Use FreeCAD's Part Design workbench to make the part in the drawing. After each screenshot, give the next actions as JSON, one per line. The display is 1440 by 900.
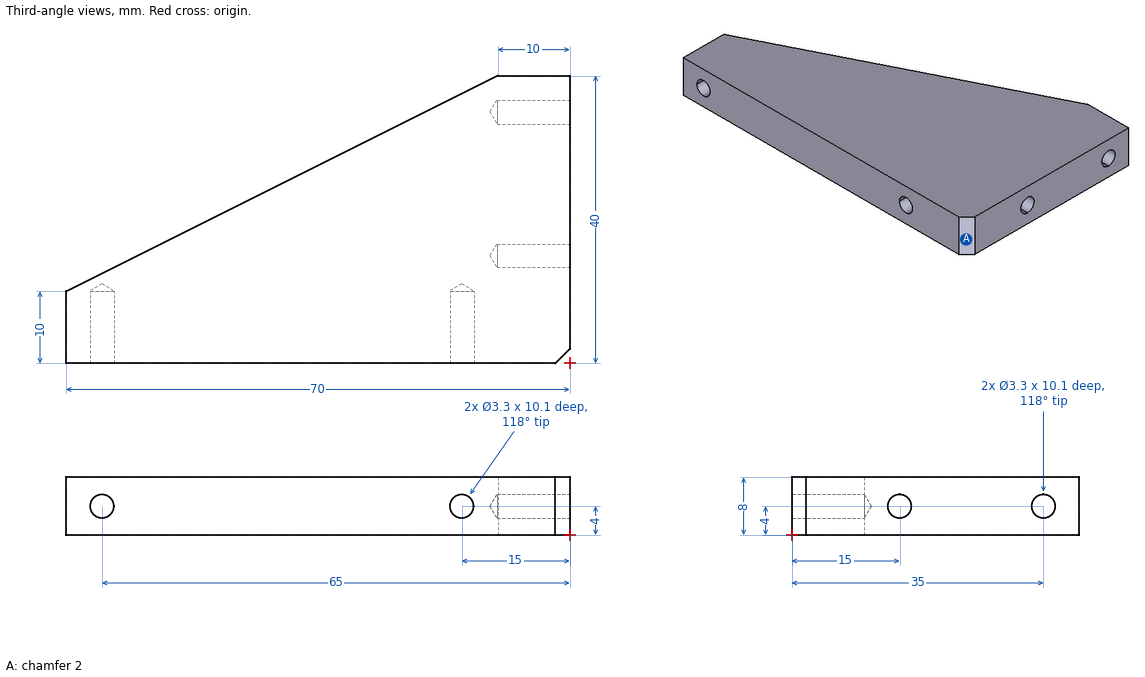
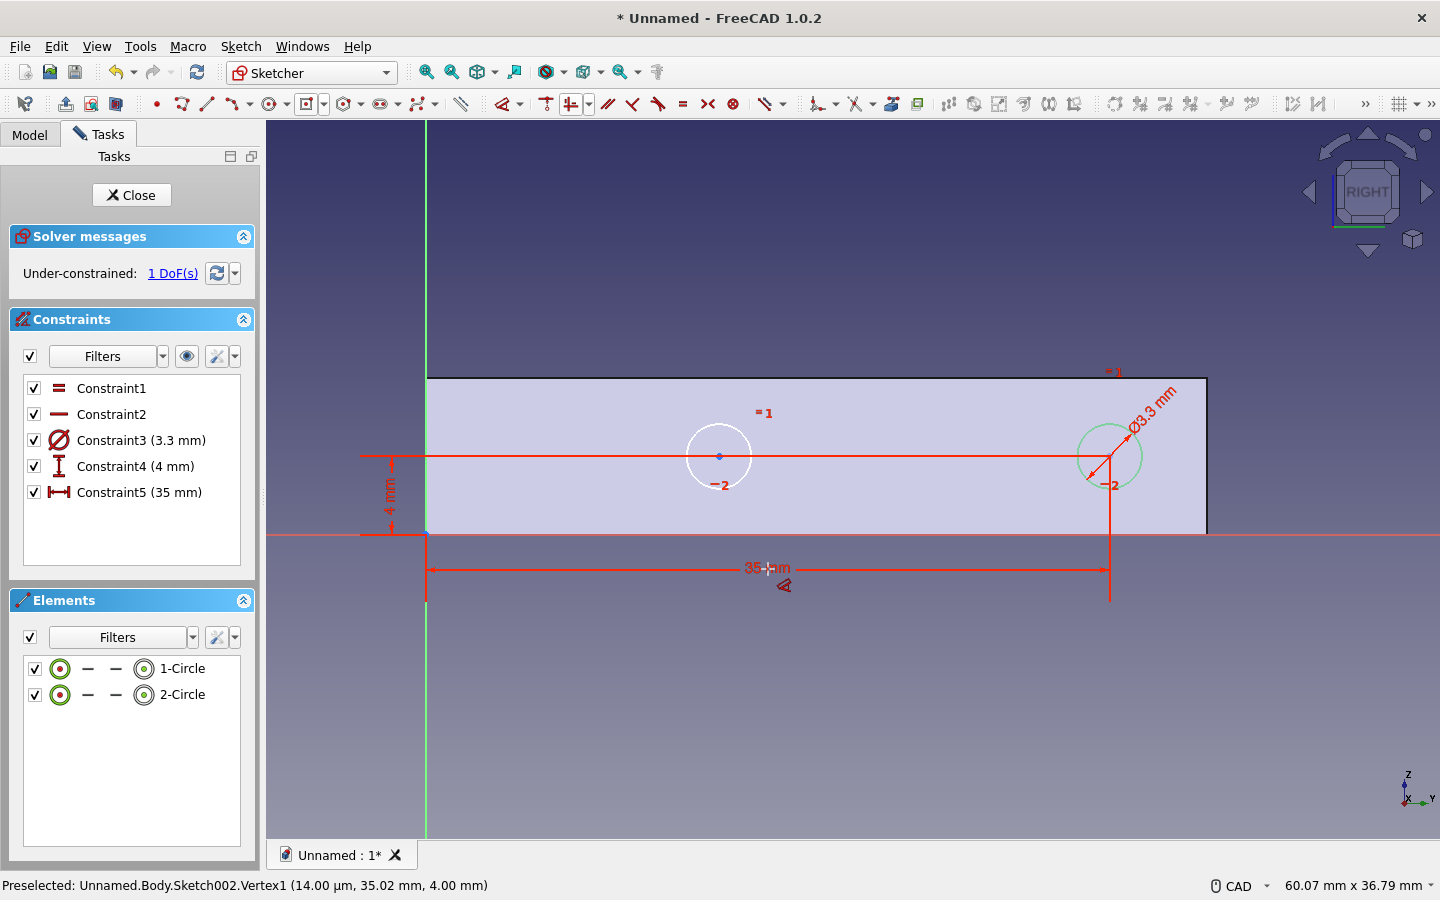
{"action": "left_click", "coordinate": [719, 456]}
{"action": "left_click", "coordinate": [572, 569]}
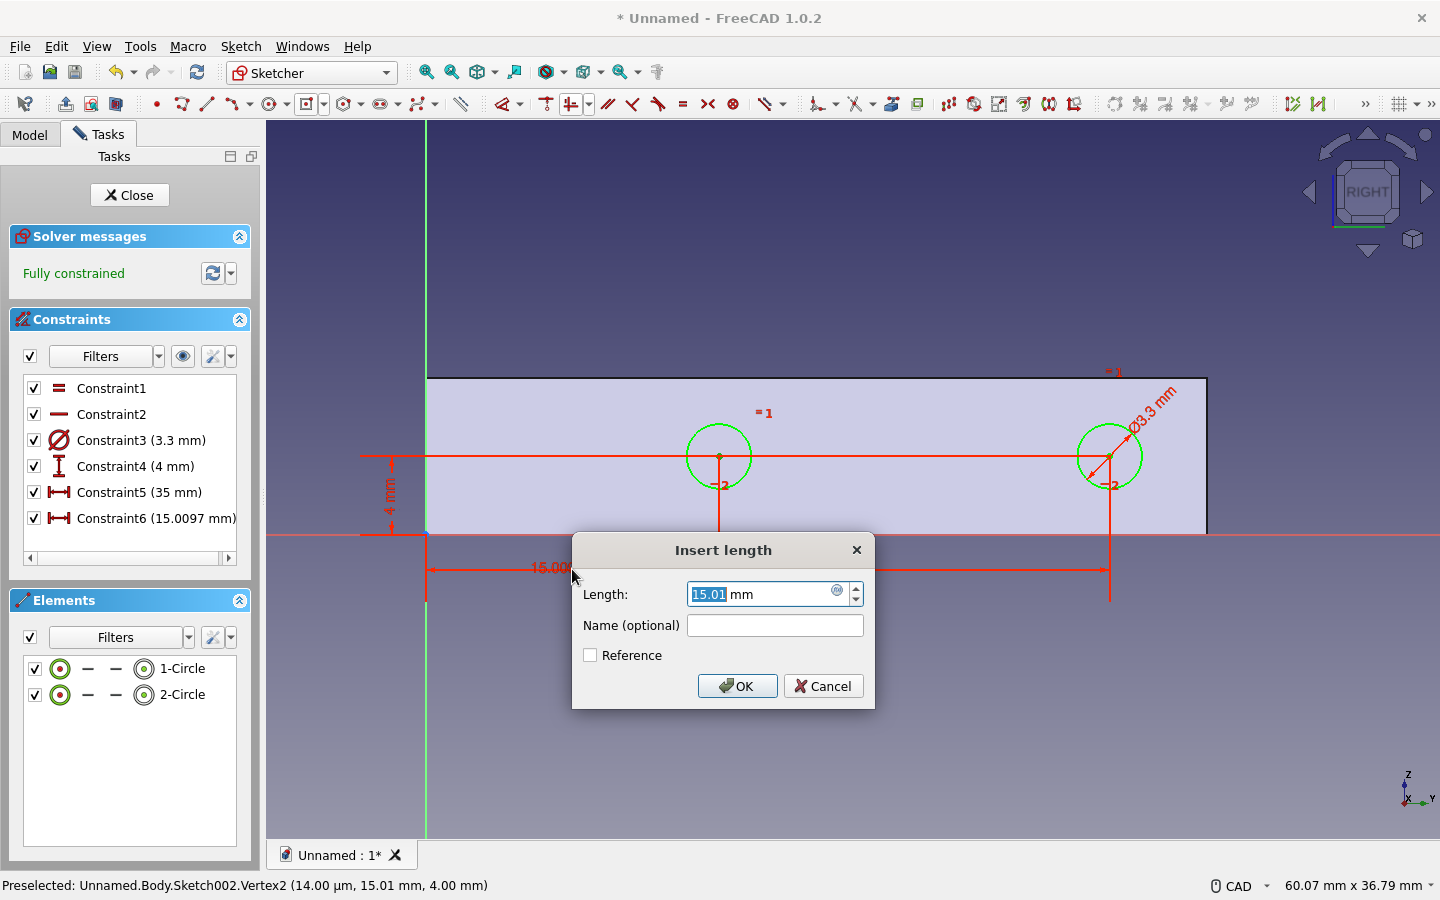
{"action": "type", "text": "15"}
{"action": "key", "text": "Return"}
{"action": "key", "text": "Escape"}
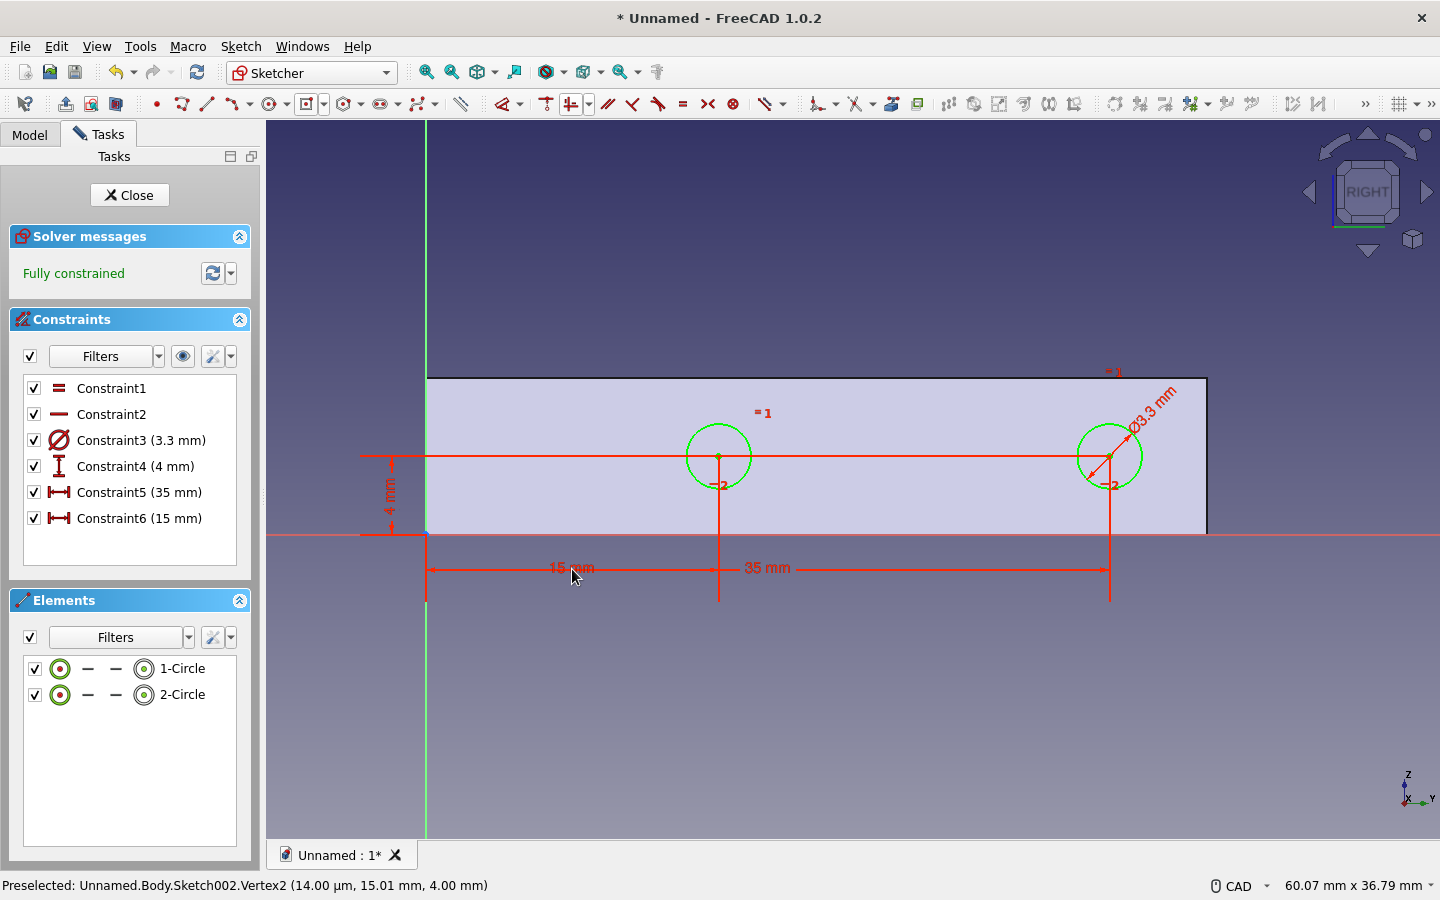
{"action": "left_click", "coordinate": [130, 195]}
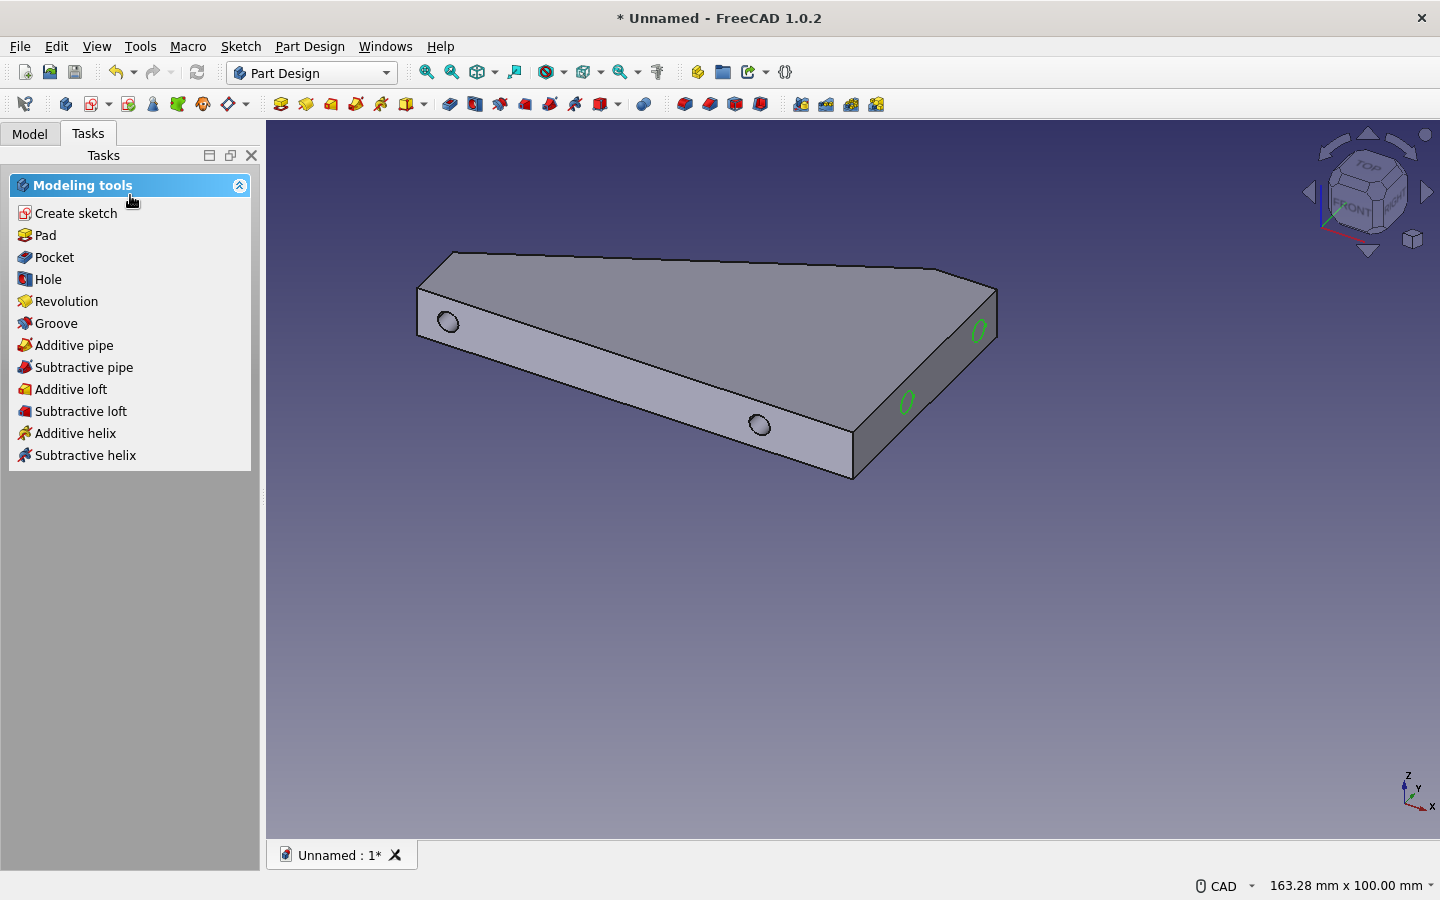
{"action": "left_click", "coordinate": [475, 104]}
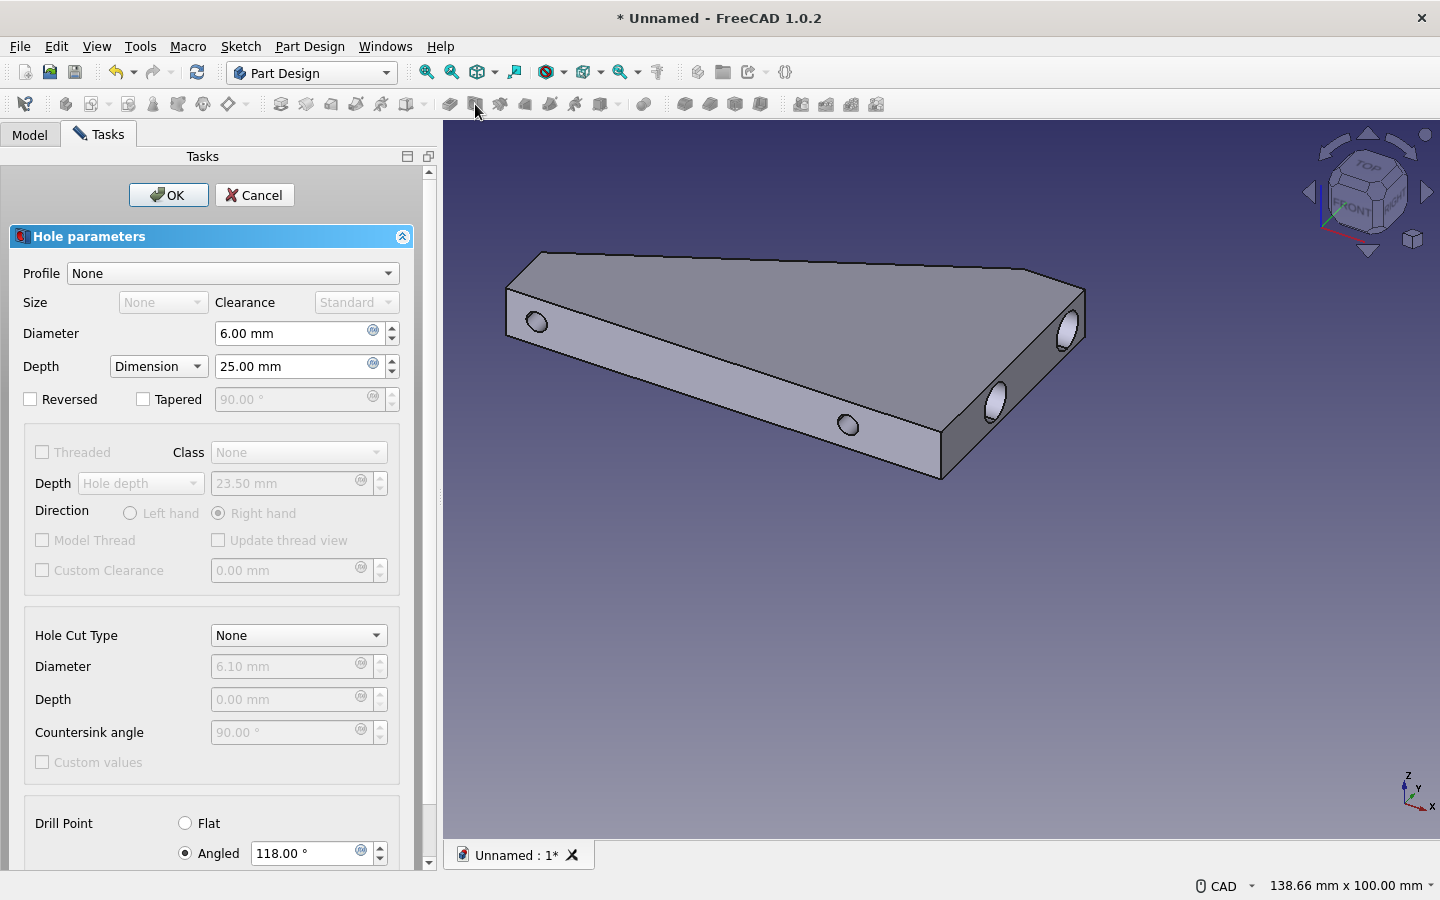
{"action": "triple_click", "coordinate": [300, 334]}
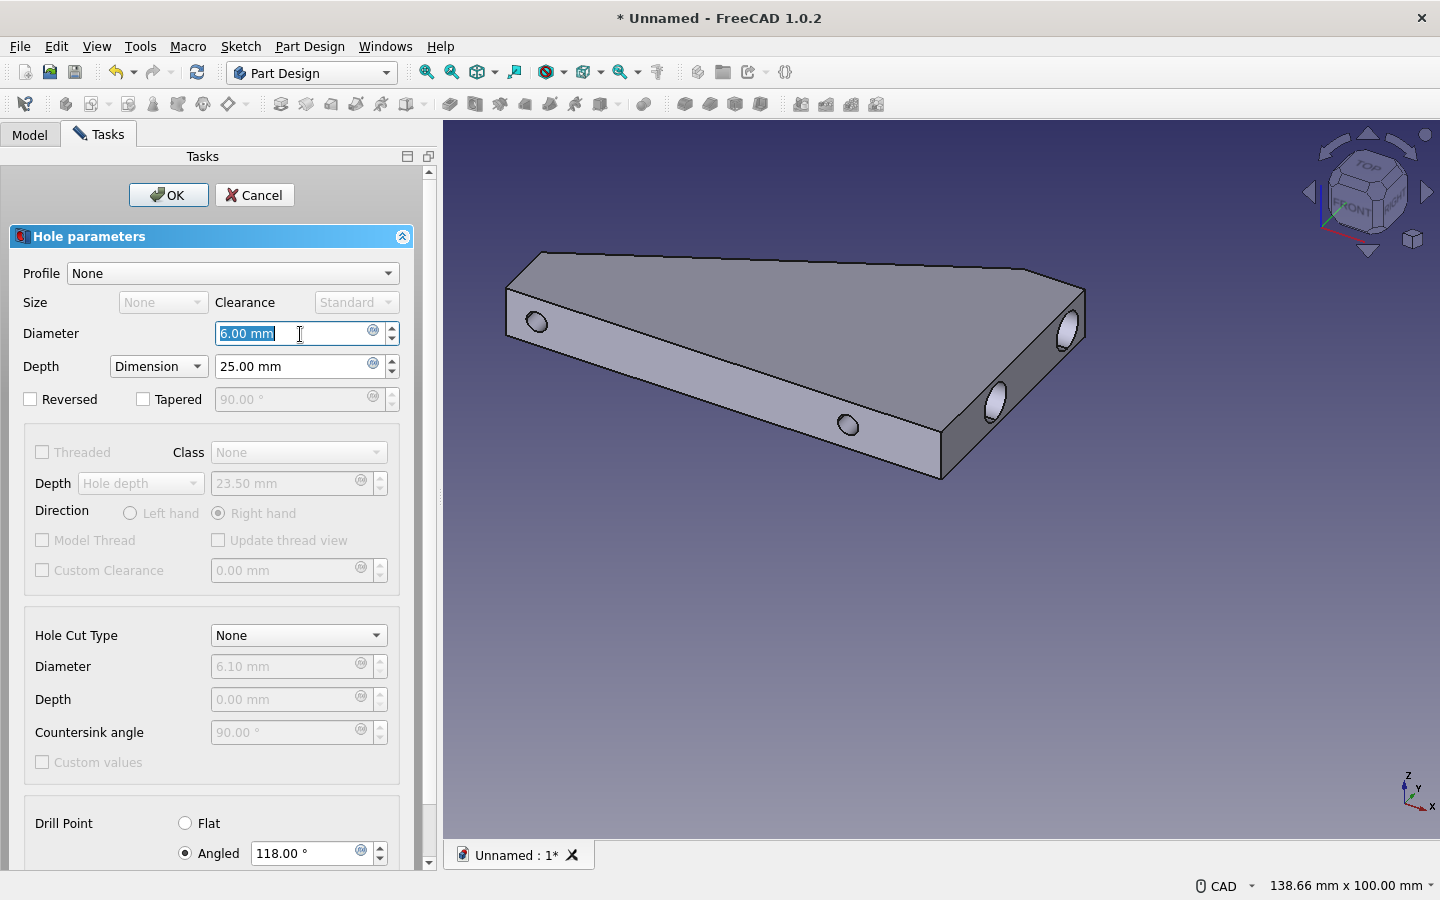
{"action": "type", "text": "3.3"}
{"action": "key", "text": "Tab"}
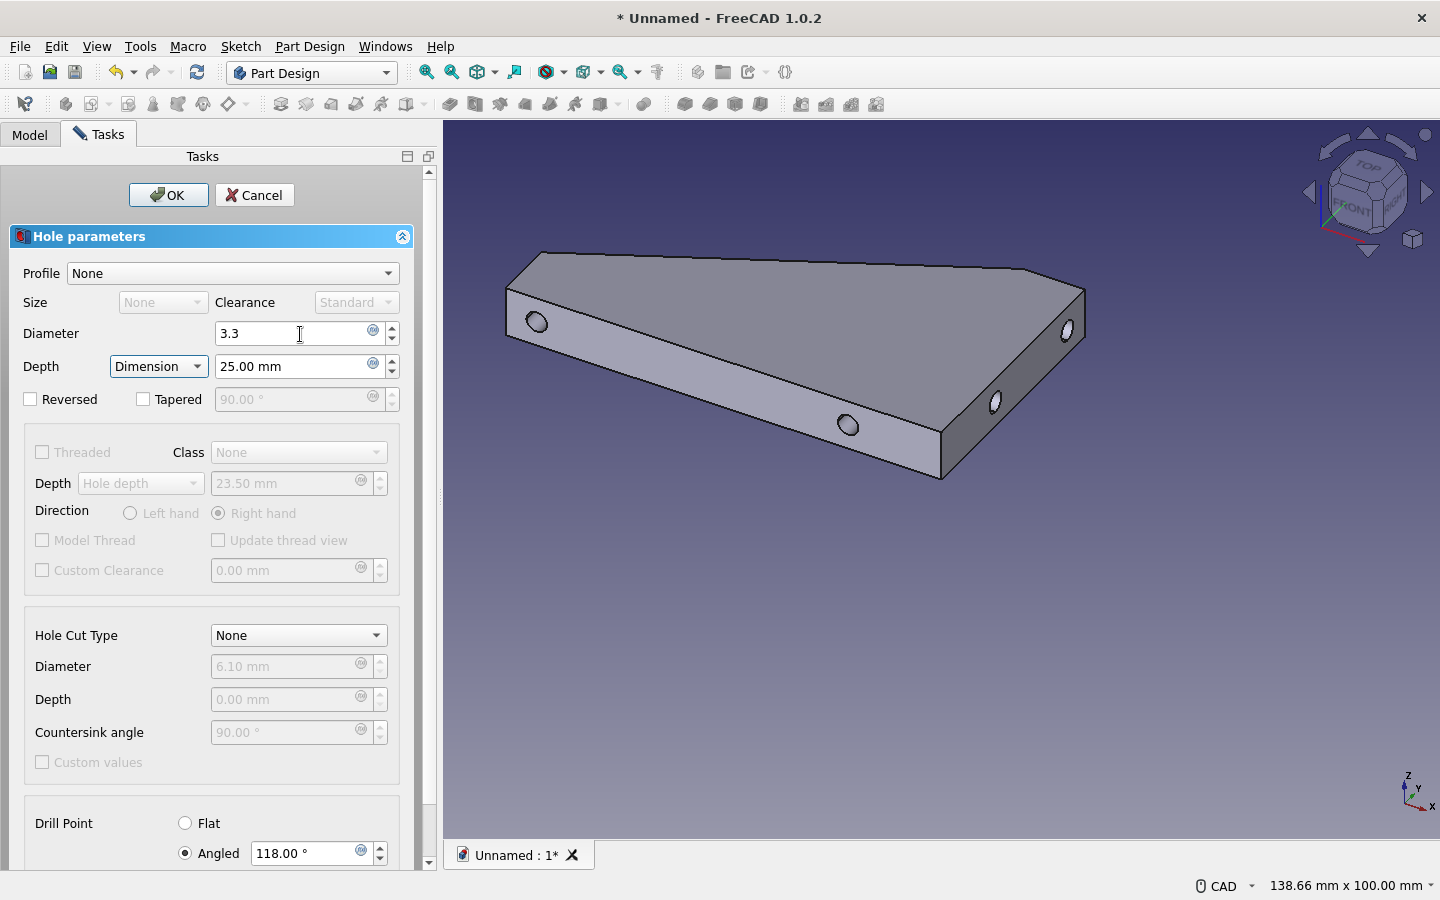
{"action": "triple_click", "coordinate": [300, 366]}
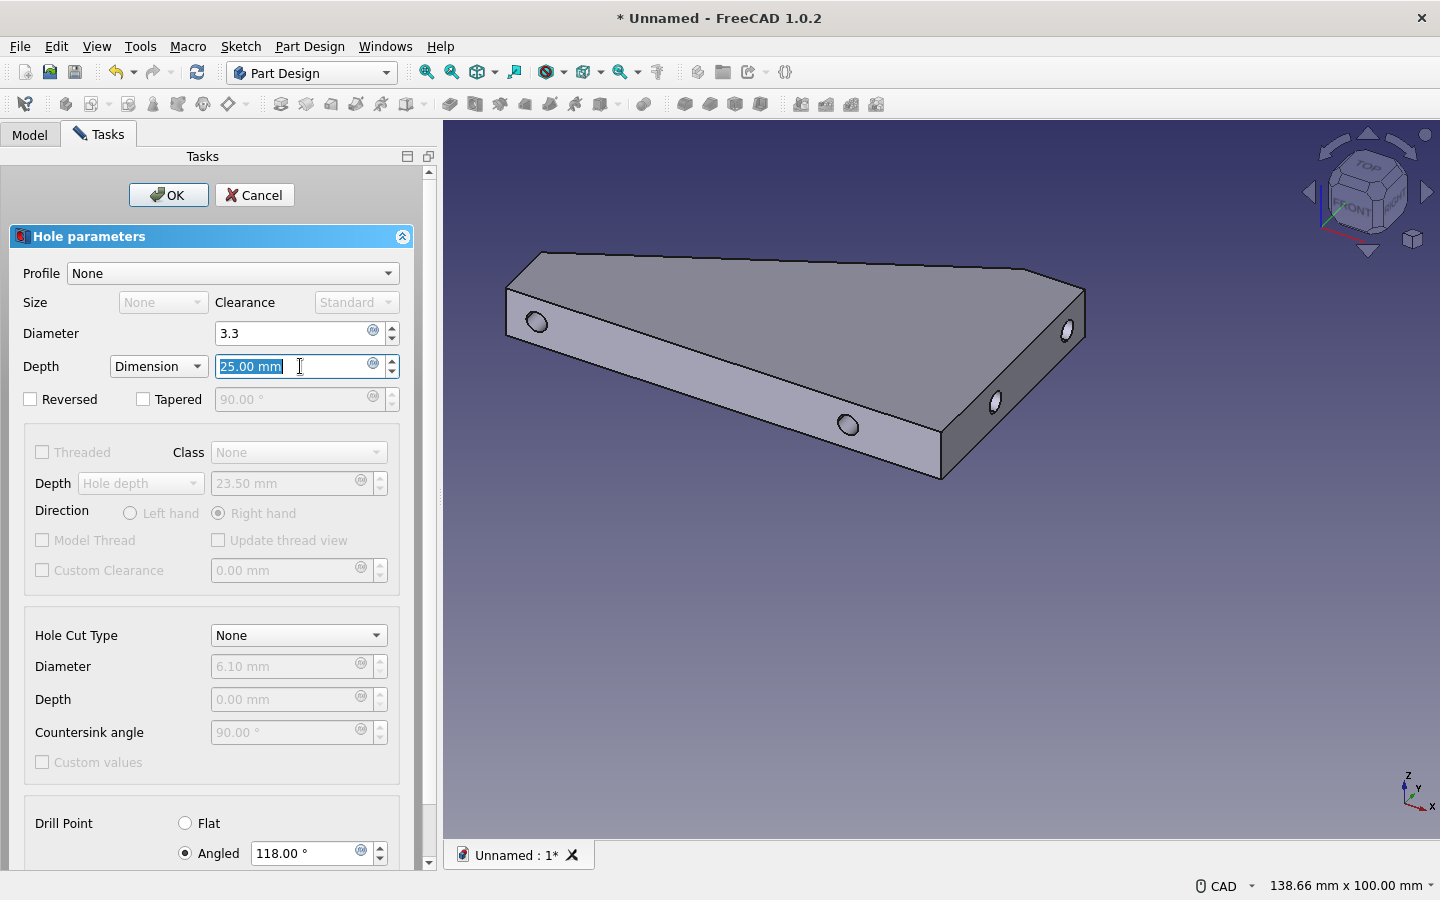
{"action": "type", "text": "10.1"}
{"action": "key", "text": "Tab"}